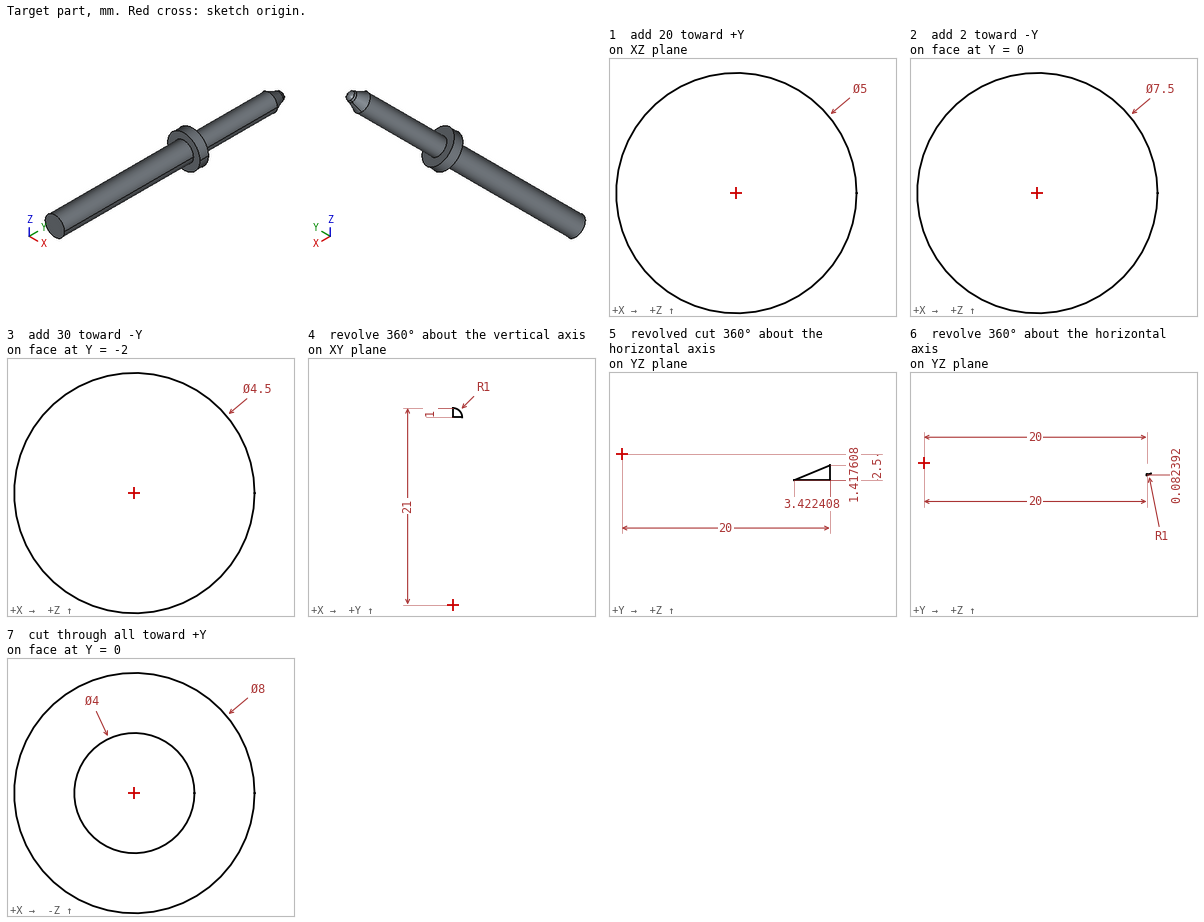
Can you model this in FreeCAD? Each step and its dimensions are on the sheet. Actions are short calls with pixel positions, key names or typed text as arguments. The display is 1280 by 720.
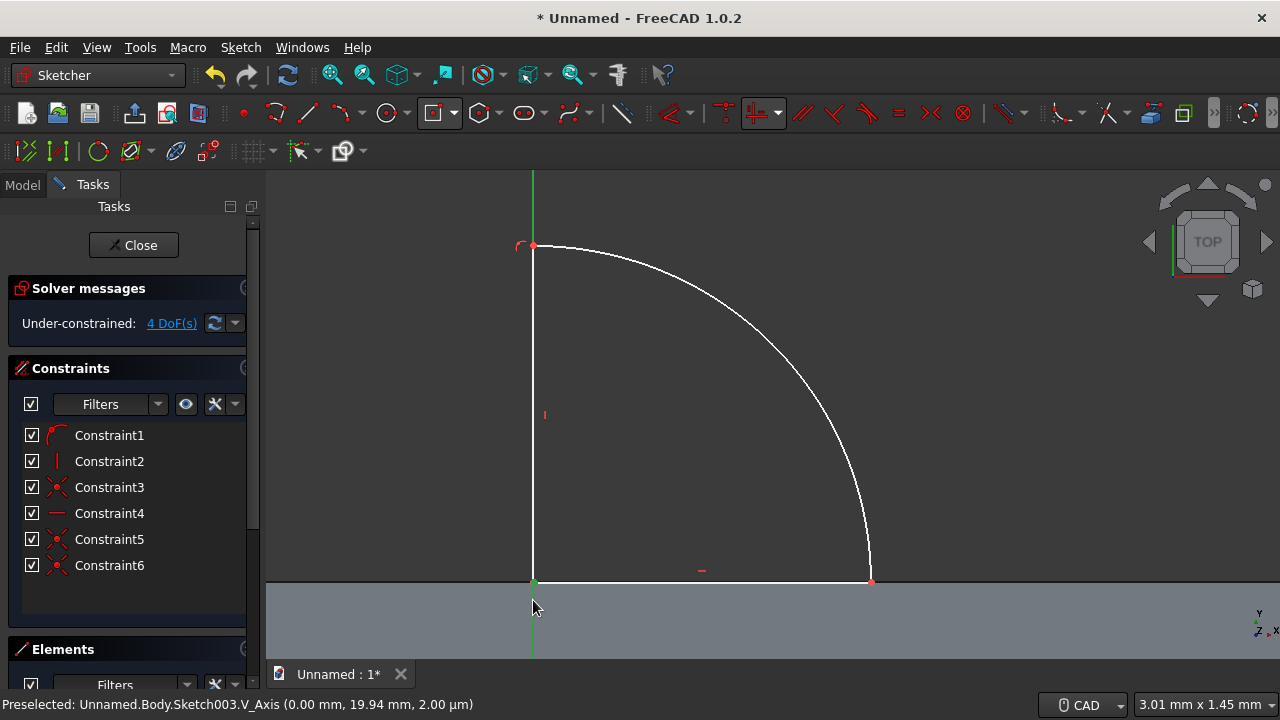
click(724, 114)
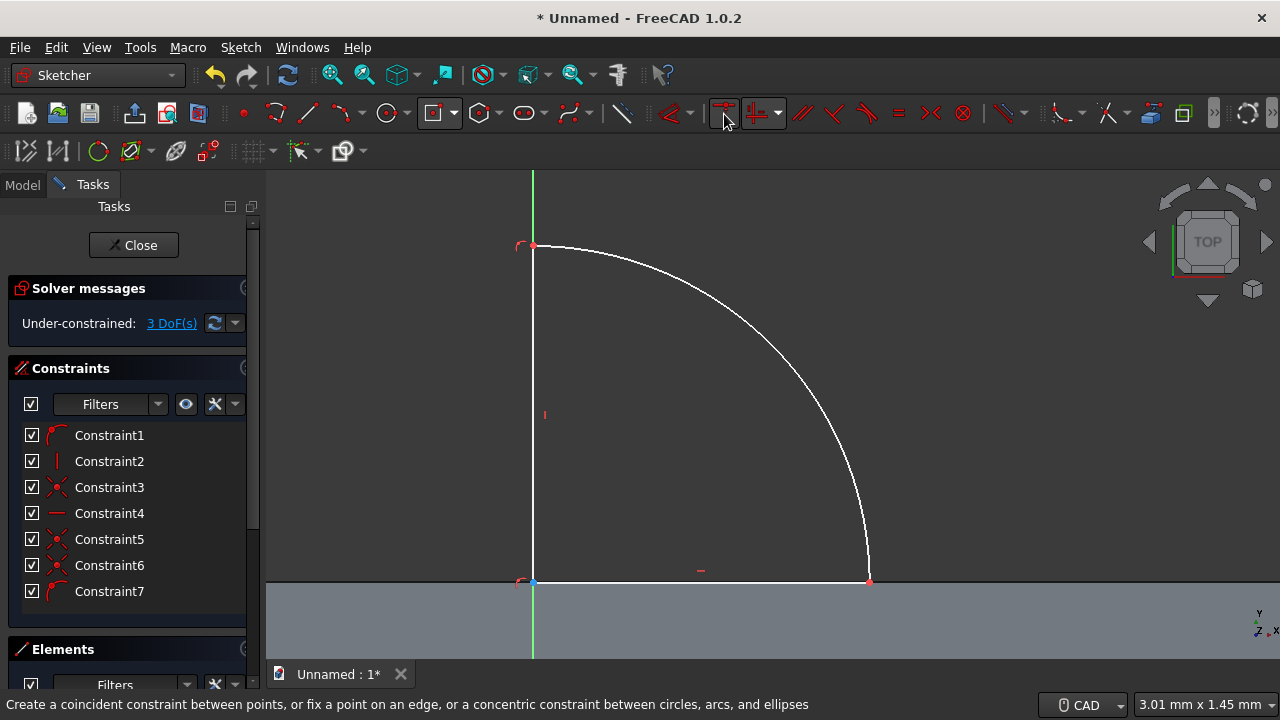
click(670, 114)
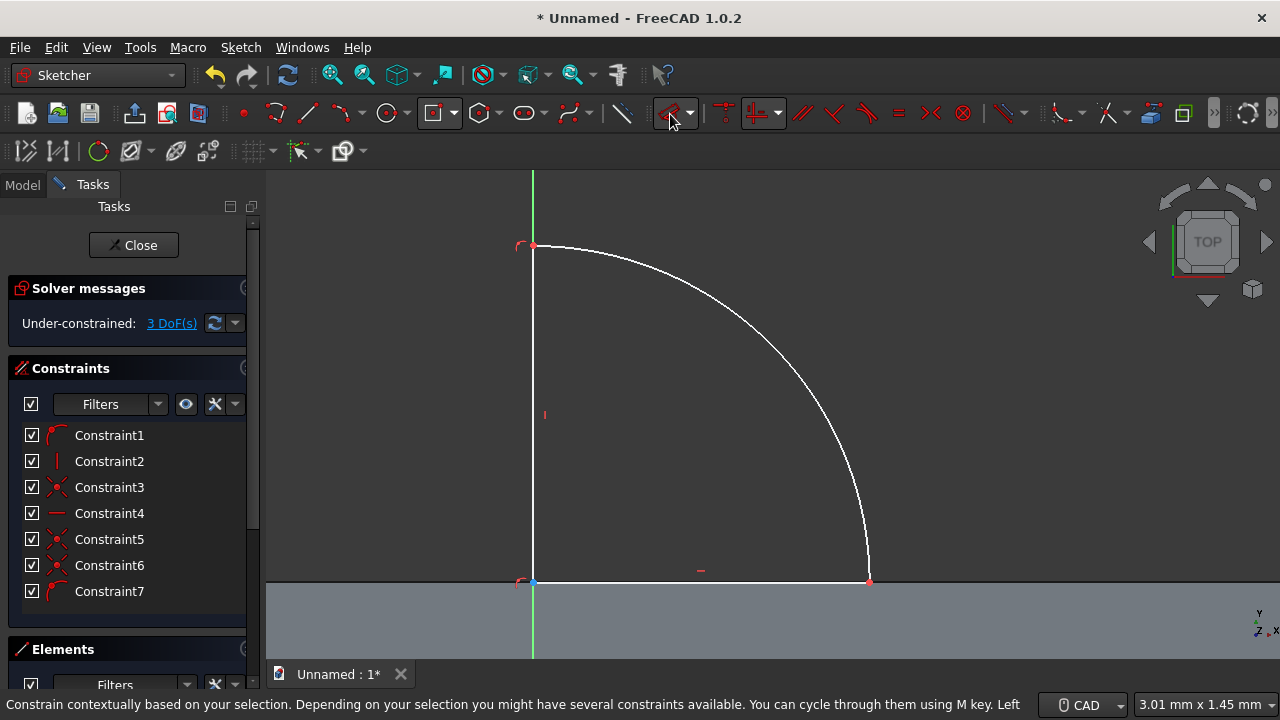
click(833, 430)
click(862, 416)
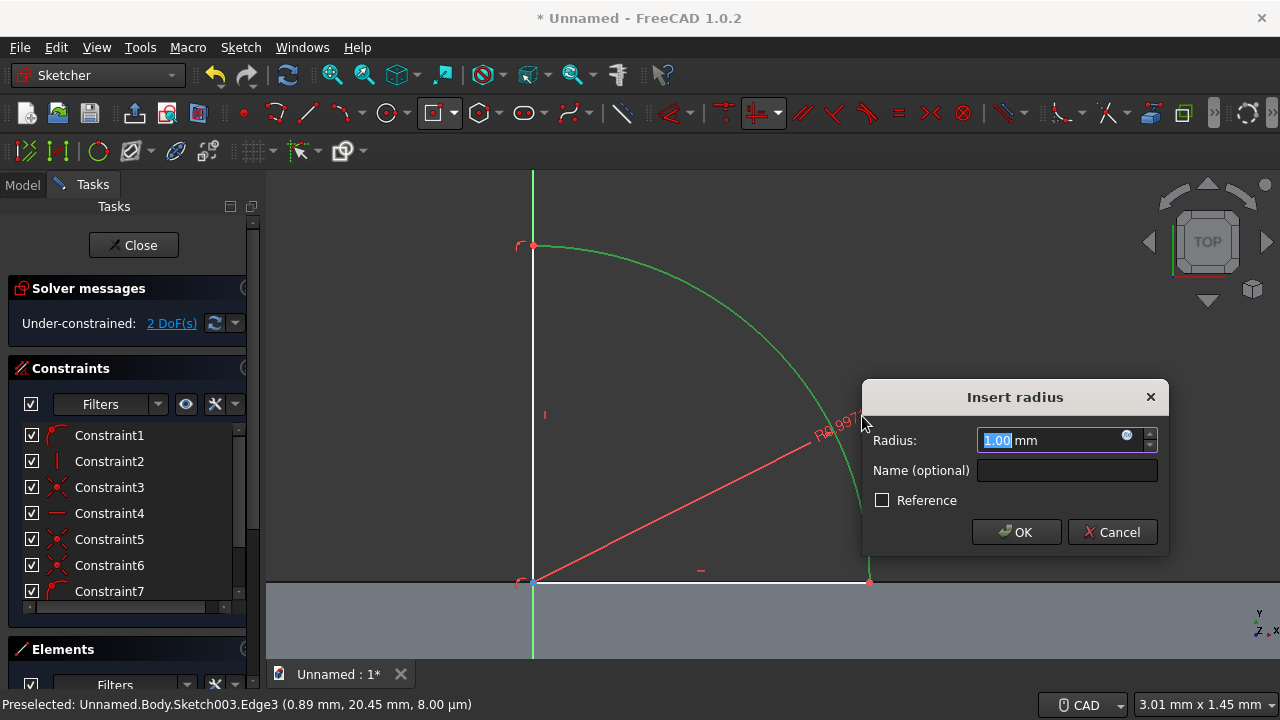
text(1)
key(Return)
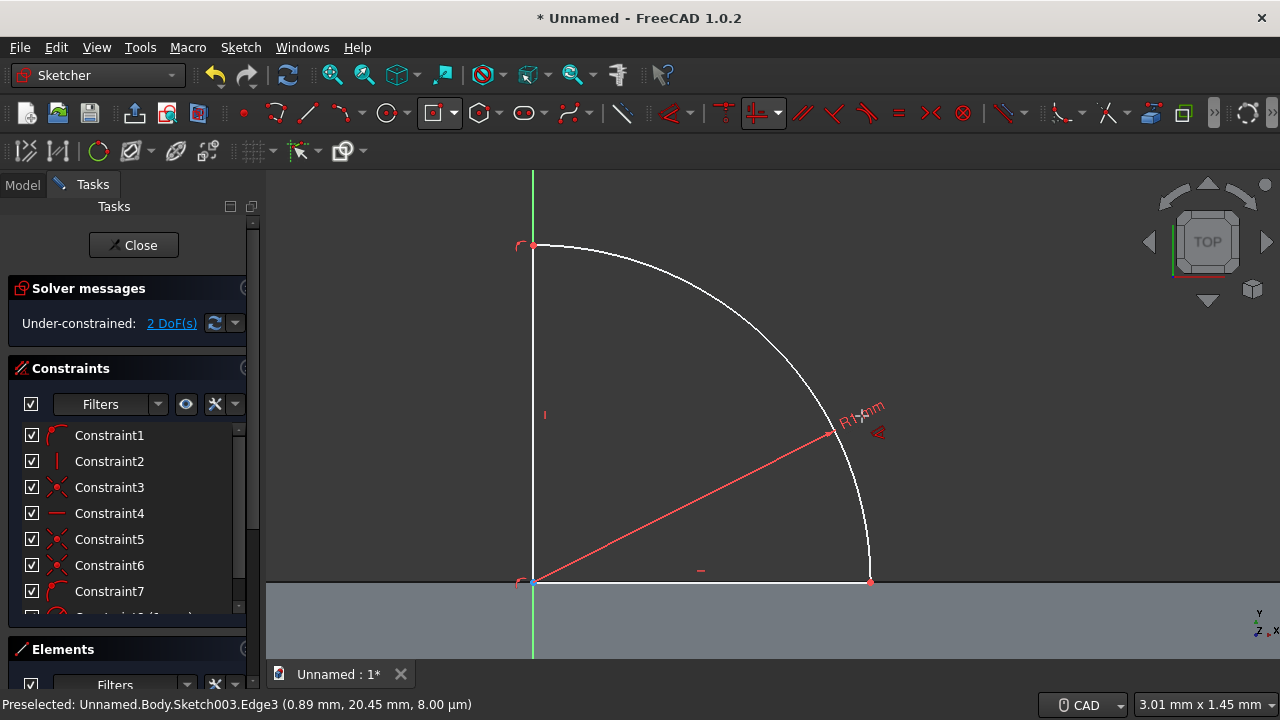
click(533, 346)
click(499, 414)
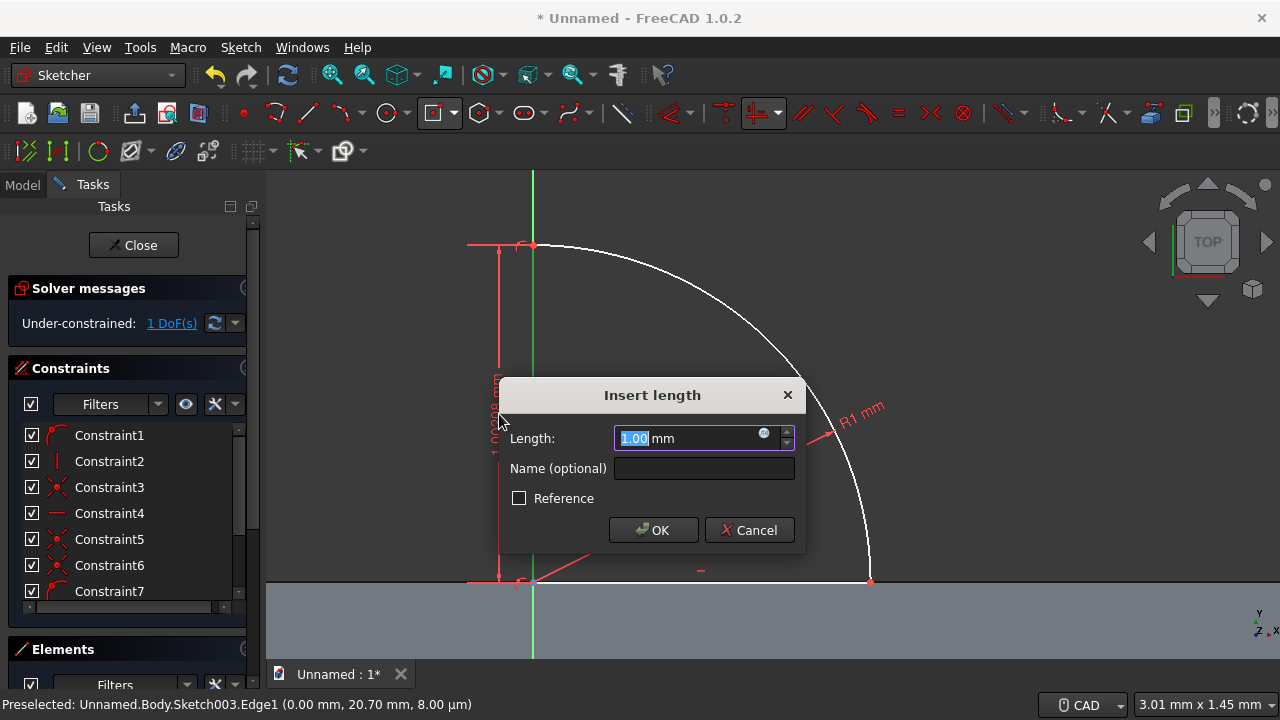
text(1)
key(Return)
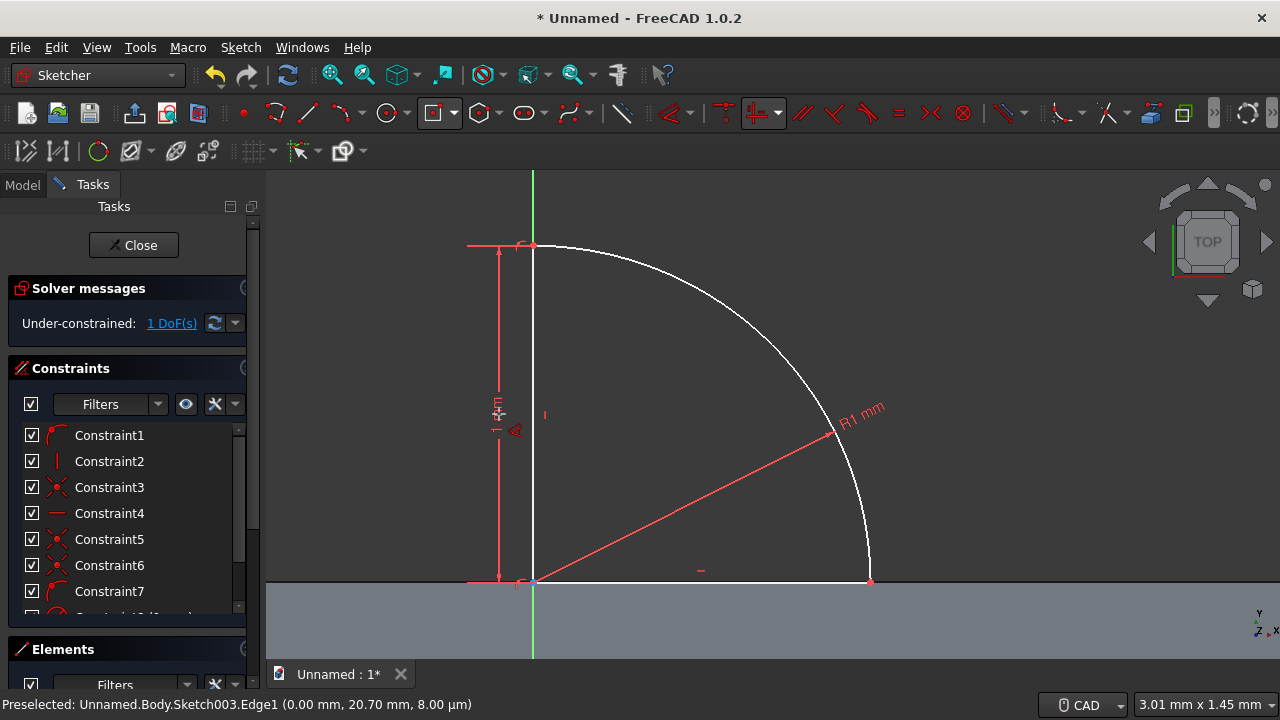
click(533, 246)
click(499, 438)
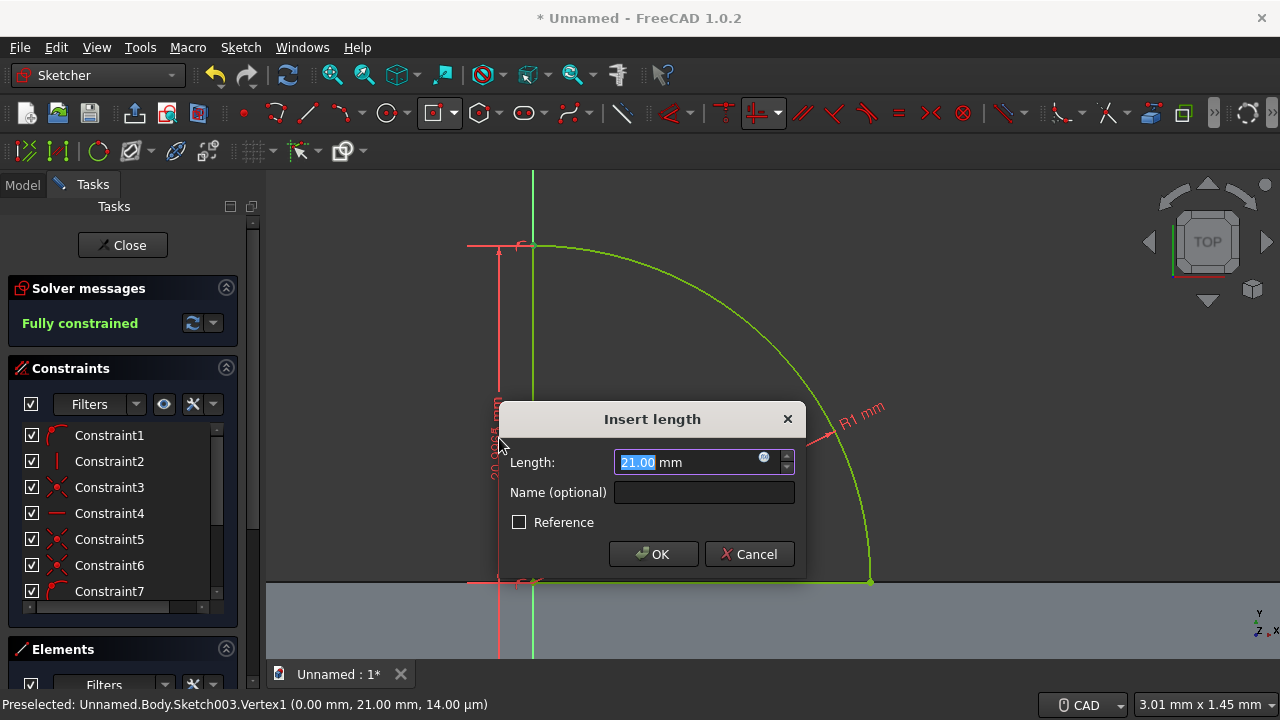
text(21)
key(Return)
key(Escape)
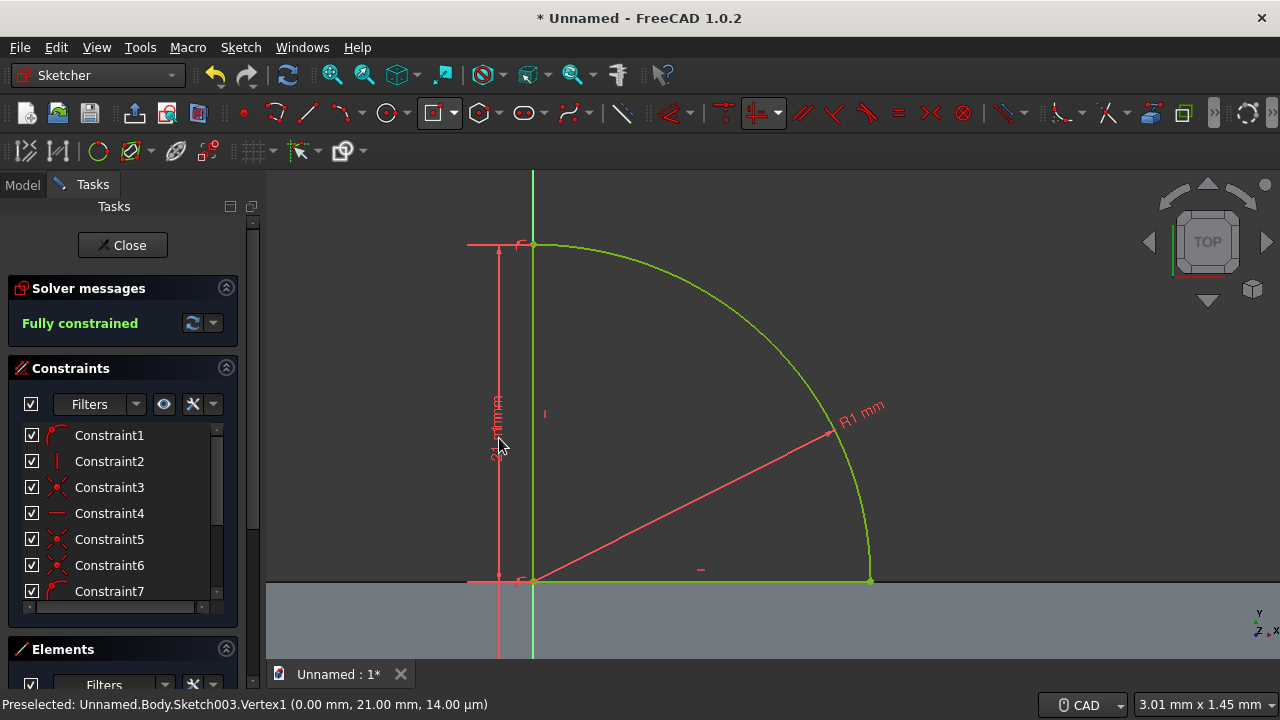
click(123, 245)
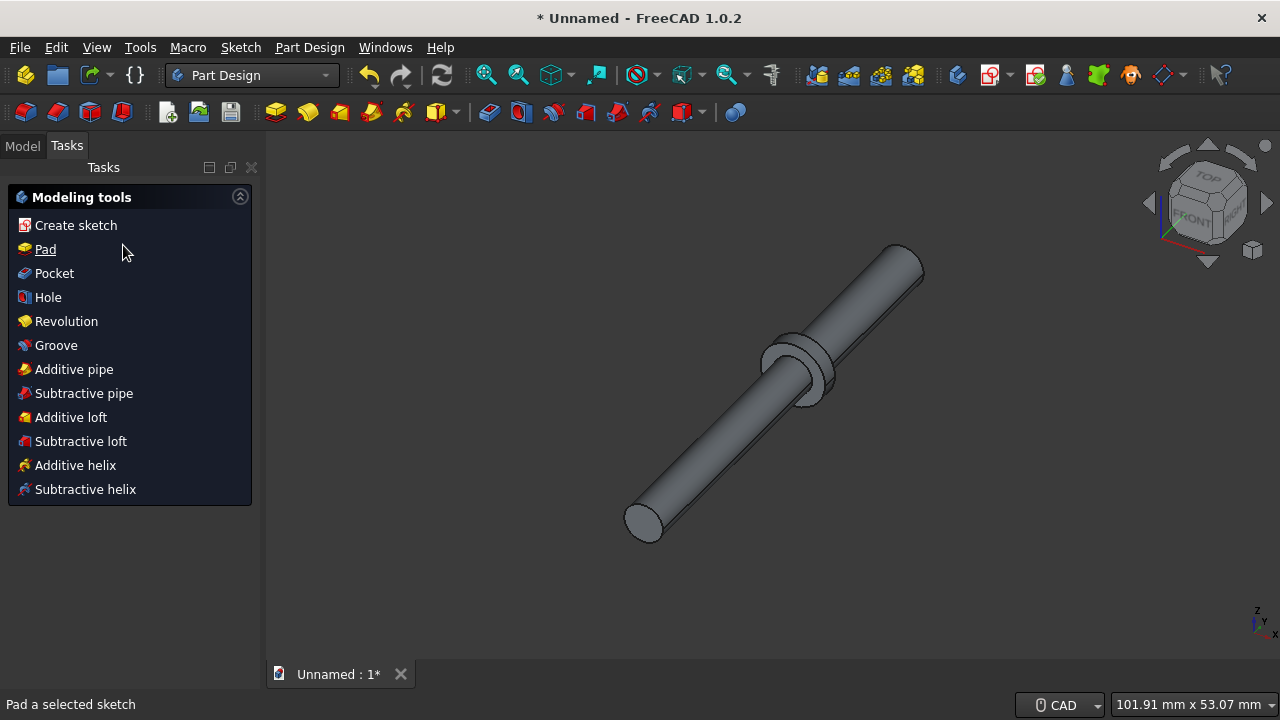
click(308, 112)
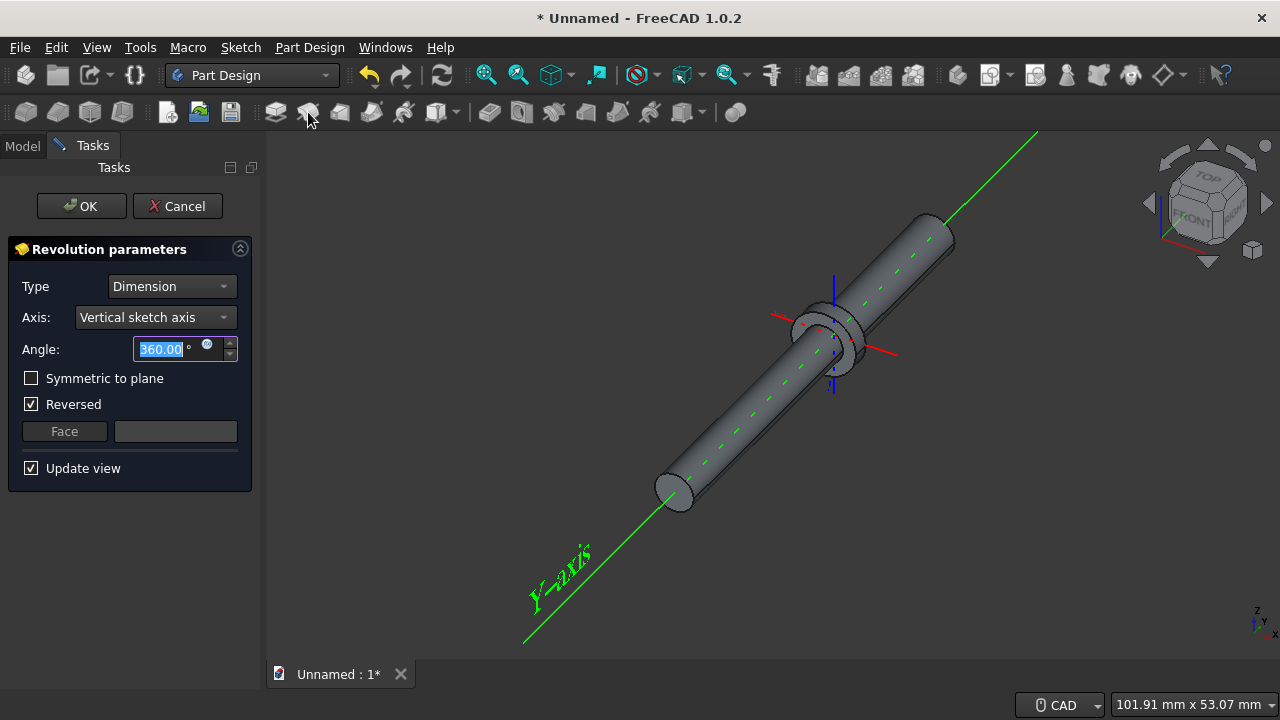
click(82, 206)